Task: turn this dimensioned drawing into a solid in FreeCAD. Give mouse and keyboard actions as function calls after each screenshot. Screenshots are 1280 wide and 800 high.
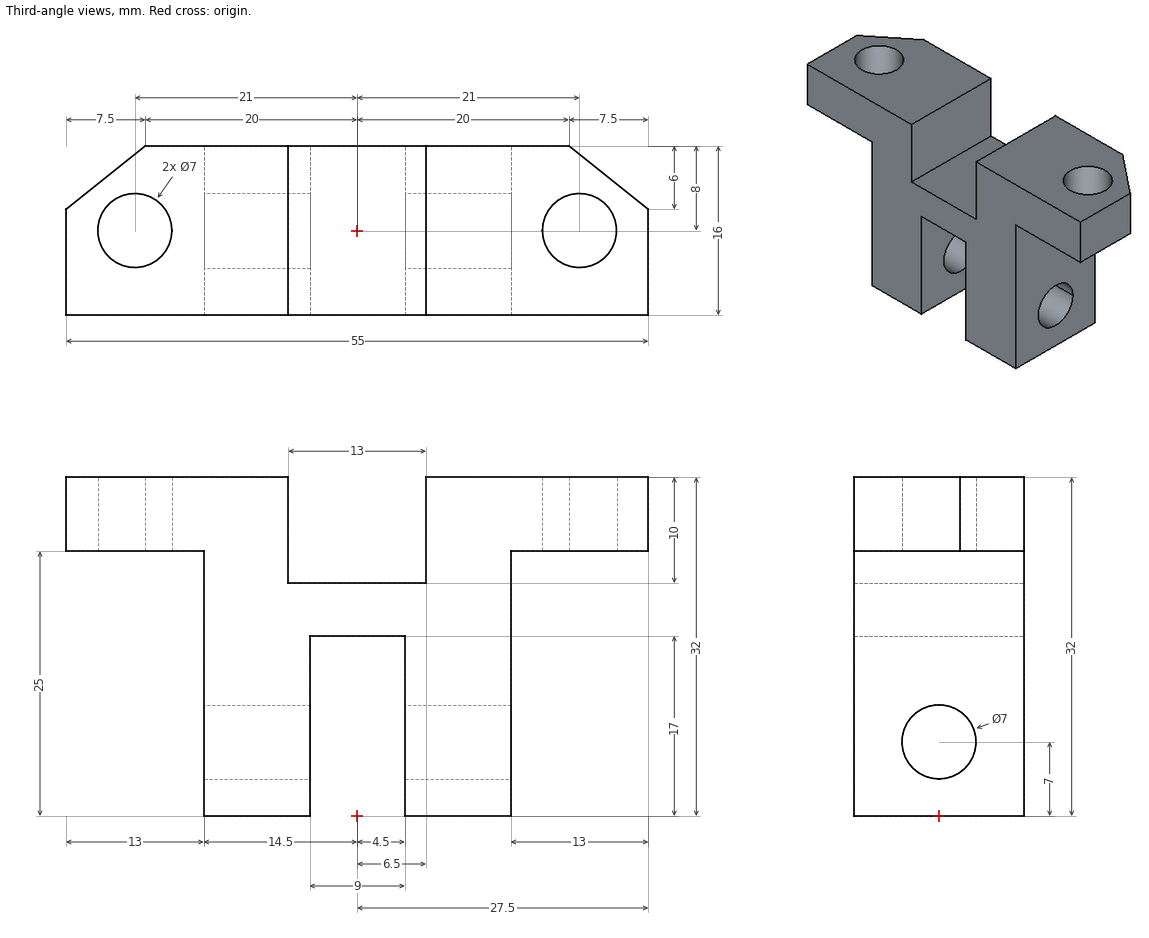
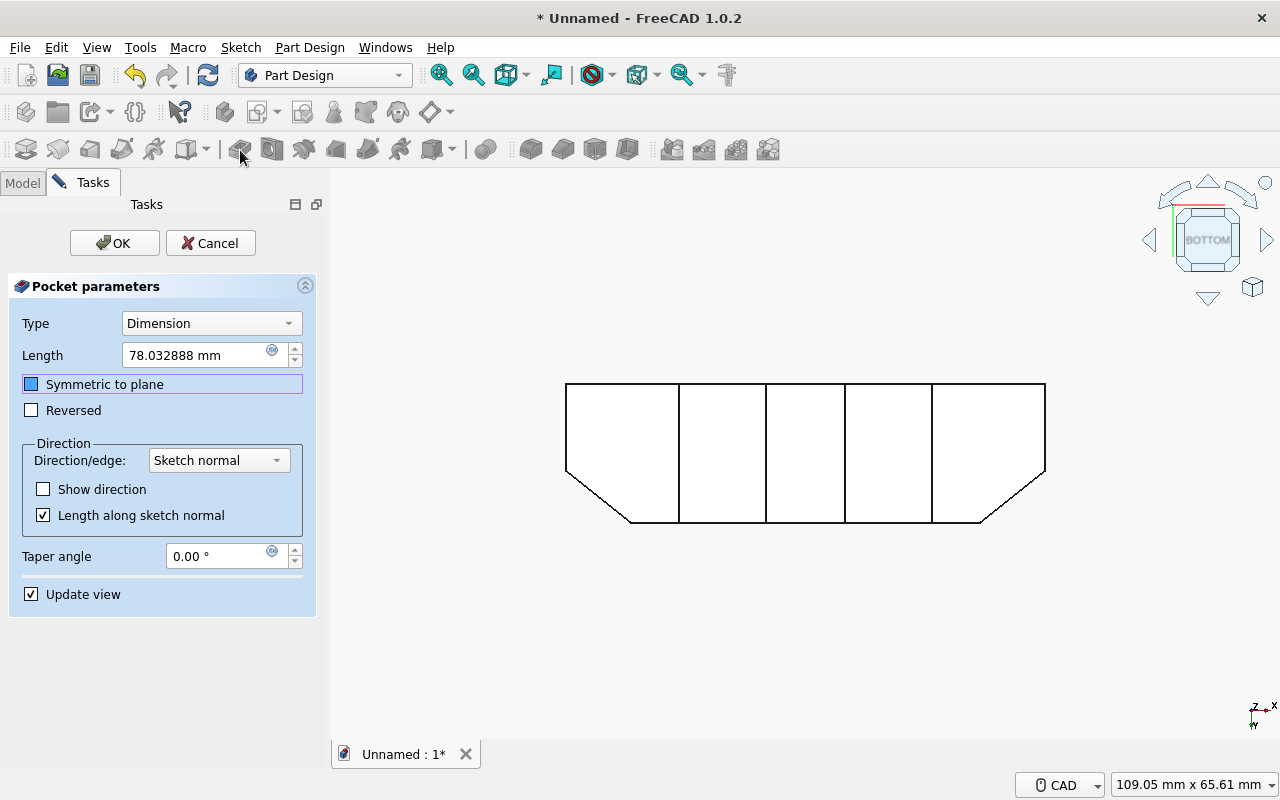
click(30, 384)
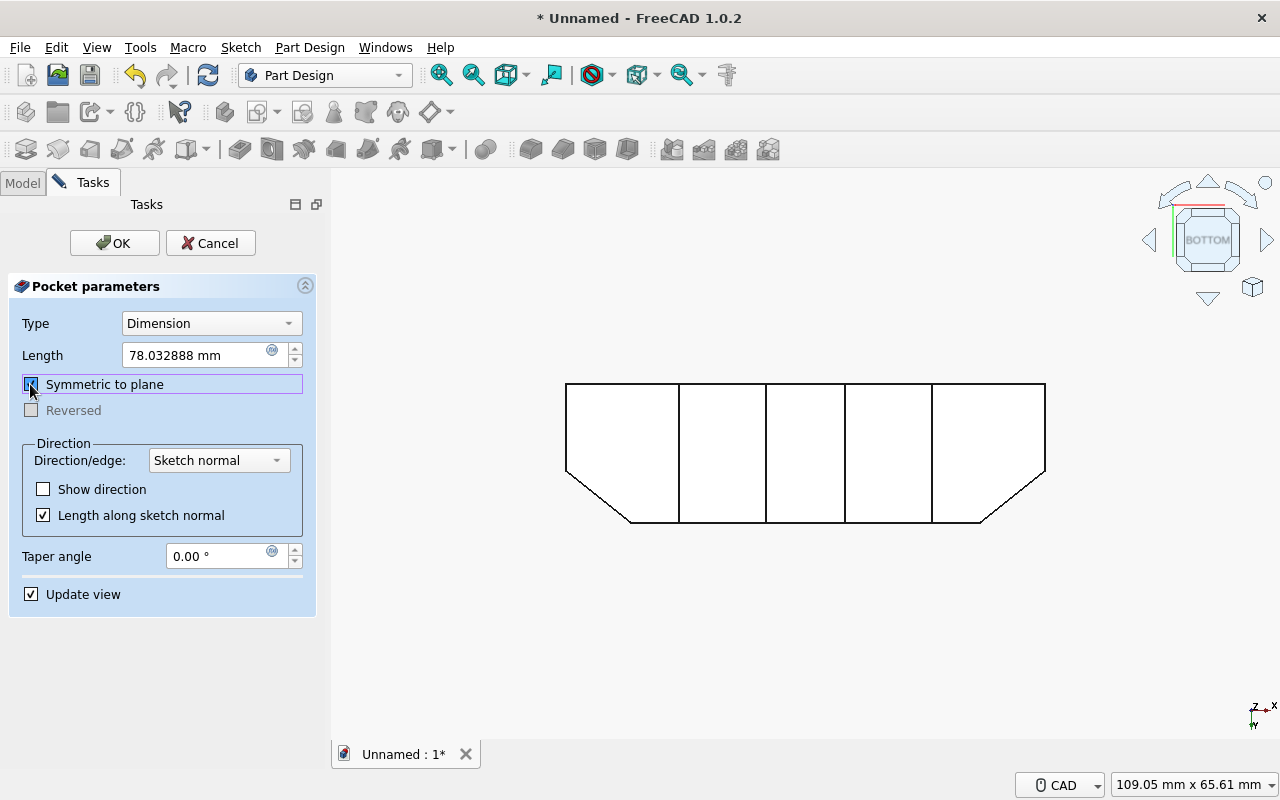
click(115, 243)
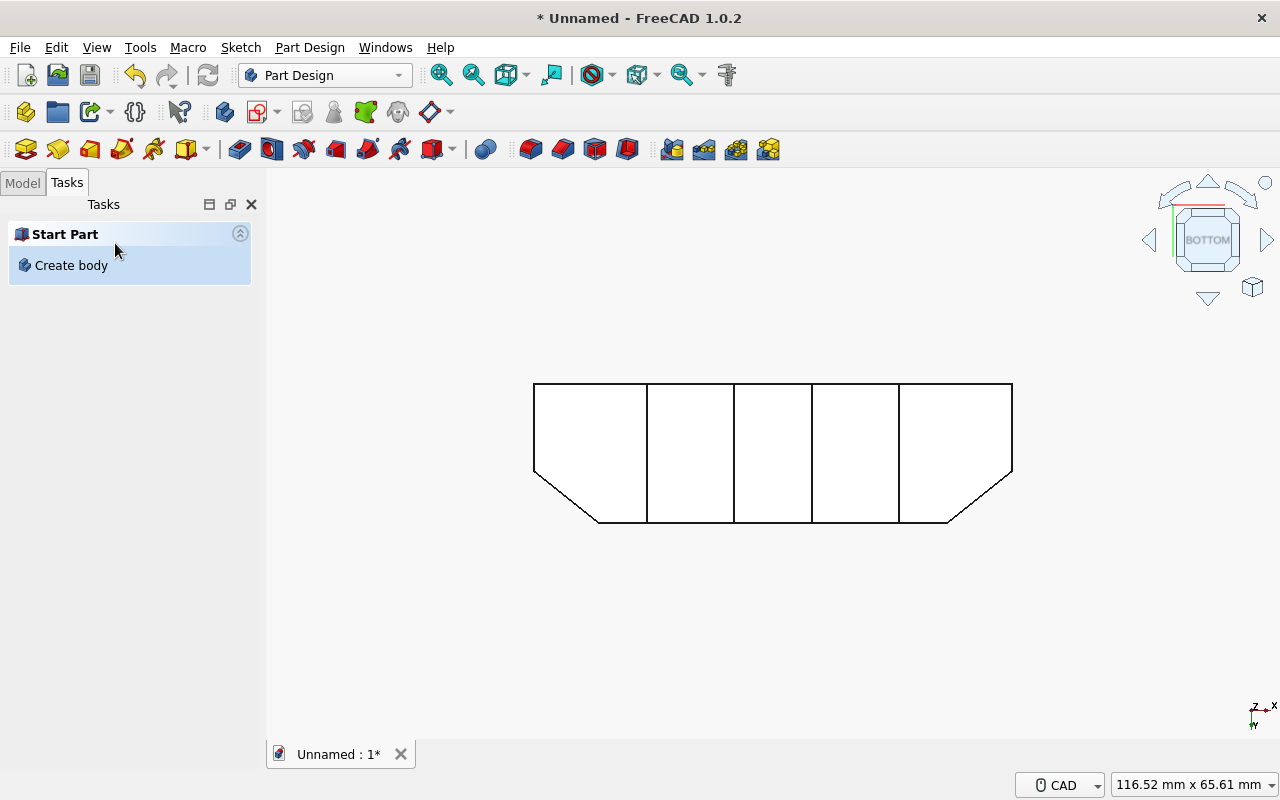
click(590, 433)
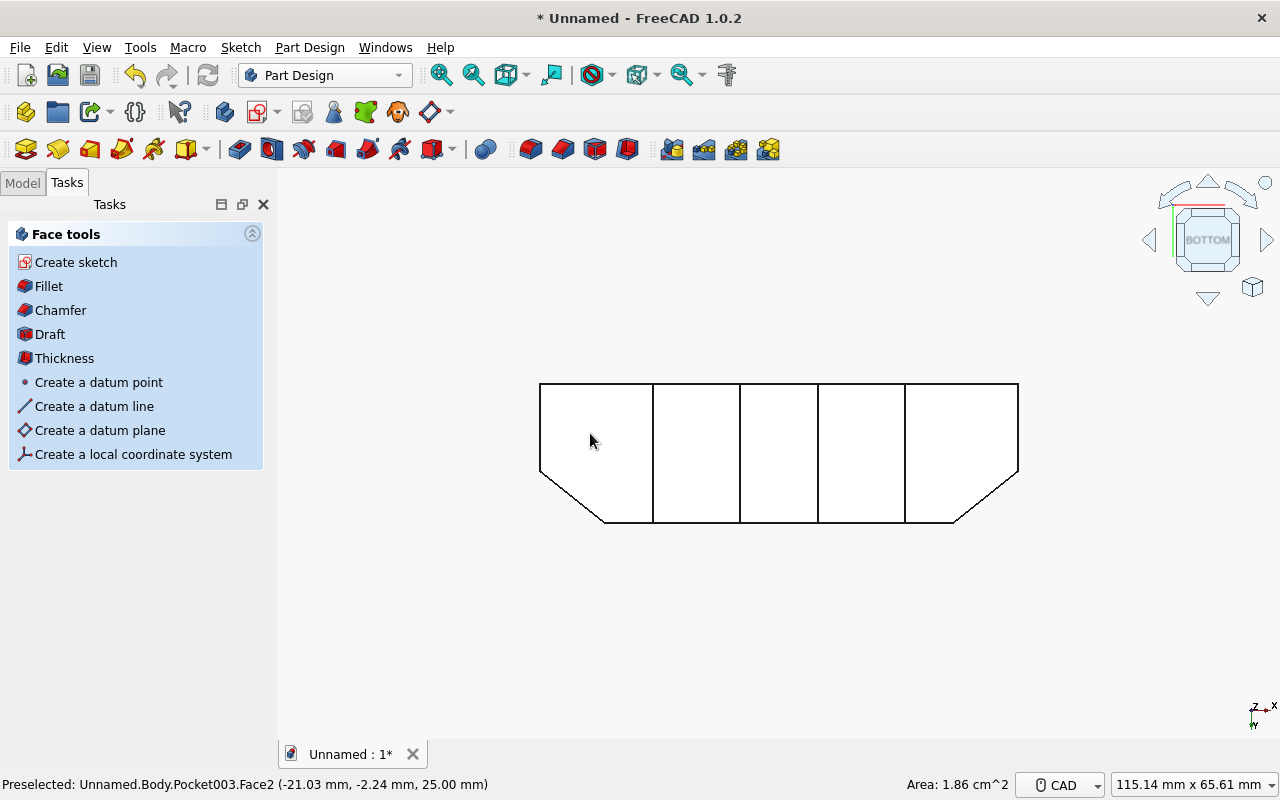
click(258, 112)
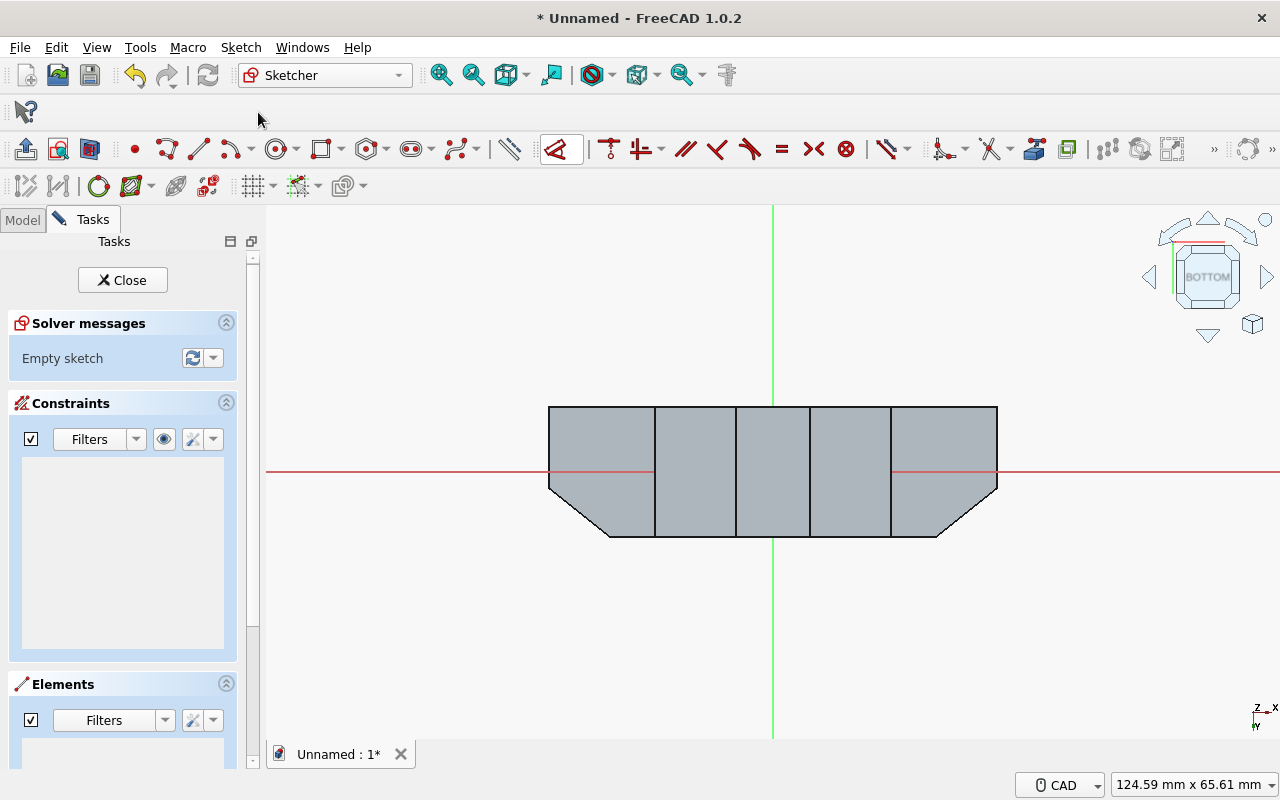
click(90, 150)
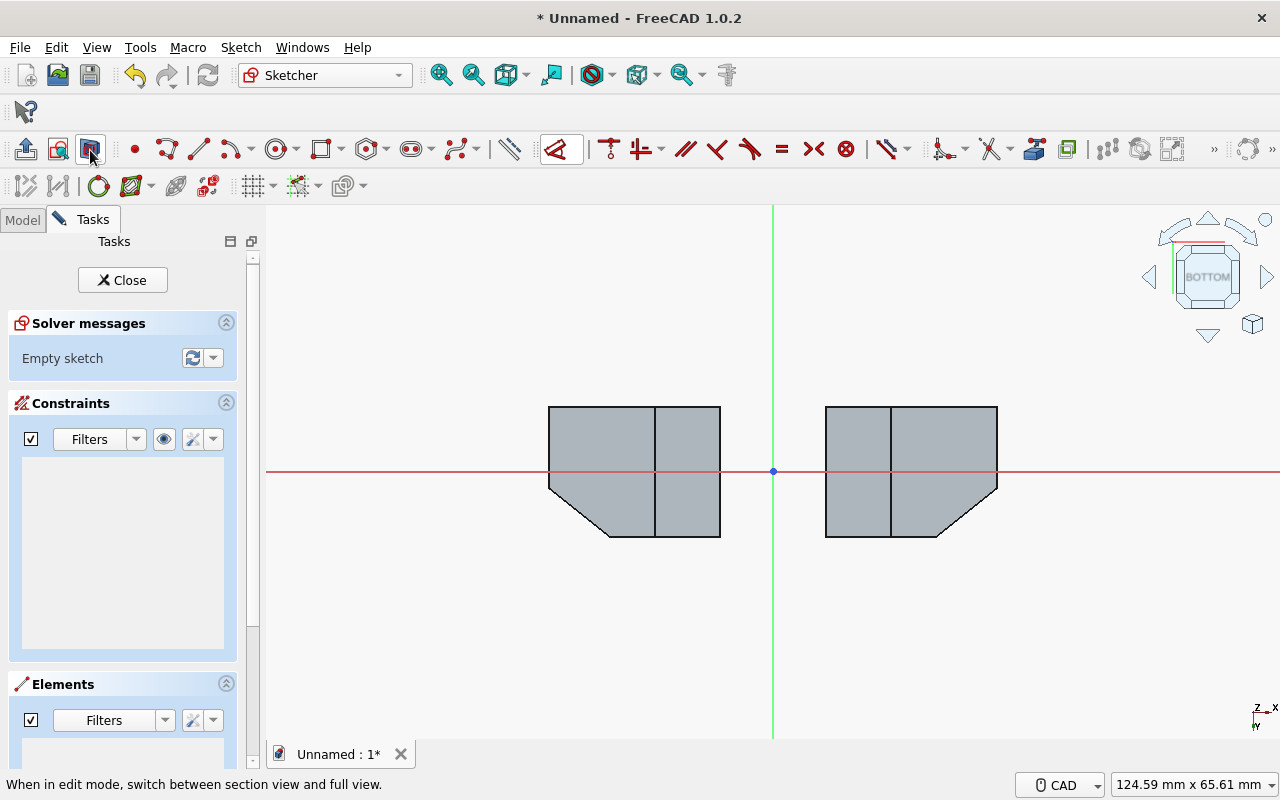
scroll(912, 472, up, 2)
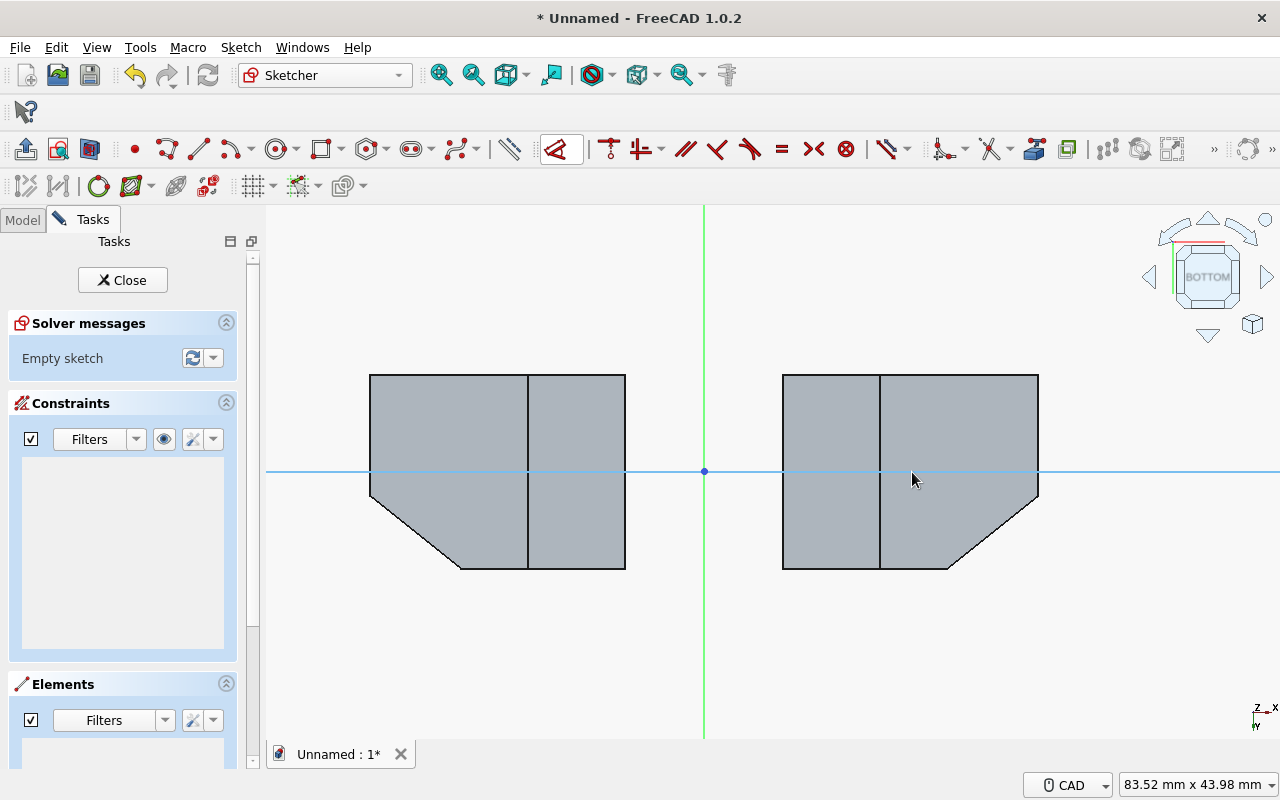
key(g)
key(c)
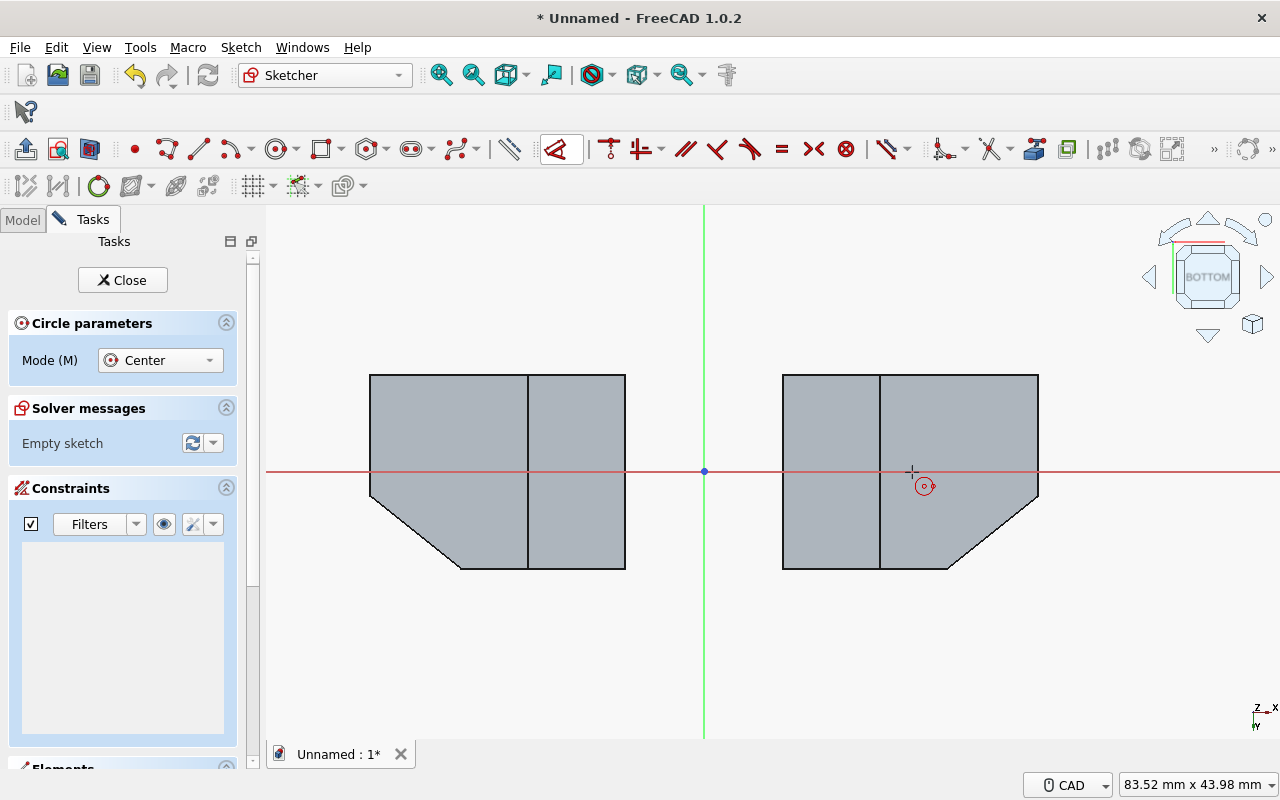
click(449, 472)
click(479, 442)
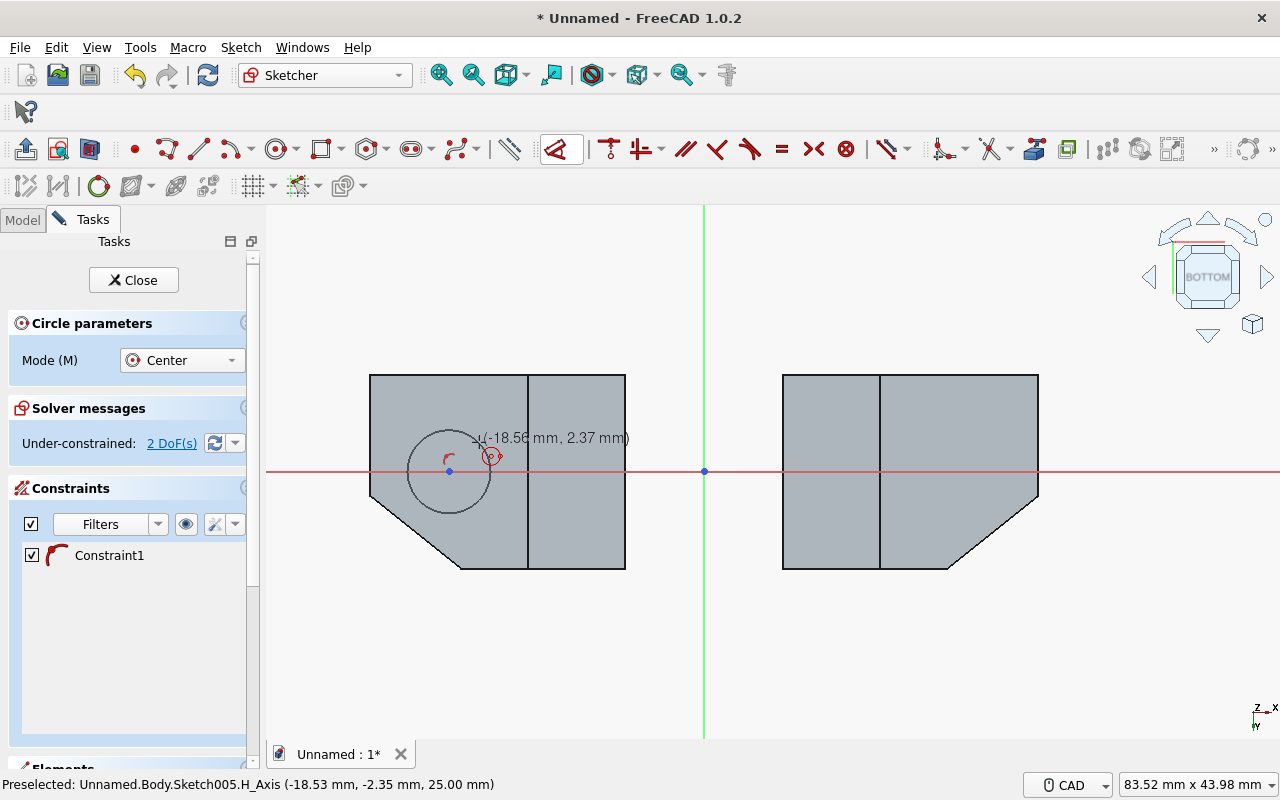
click(959, 472)
click(989, 442)
key(Escape)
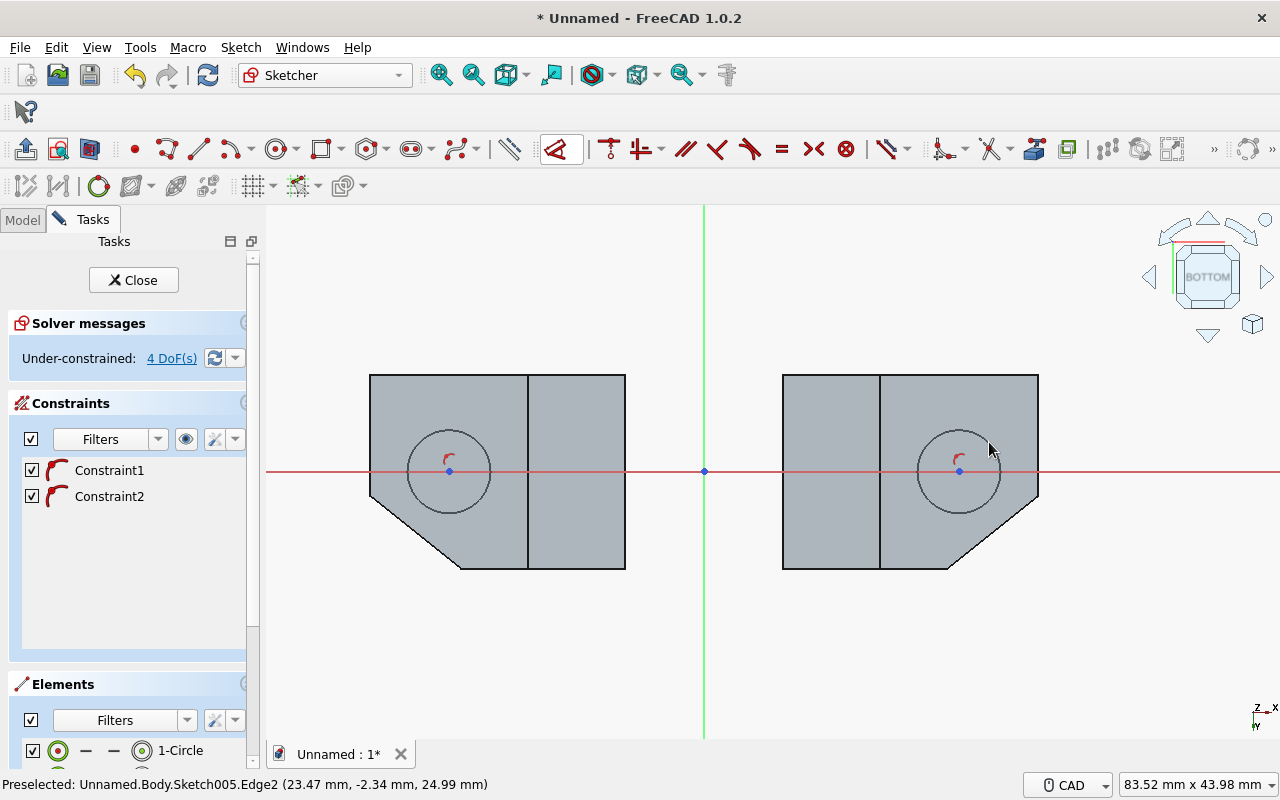
click(478, 442)